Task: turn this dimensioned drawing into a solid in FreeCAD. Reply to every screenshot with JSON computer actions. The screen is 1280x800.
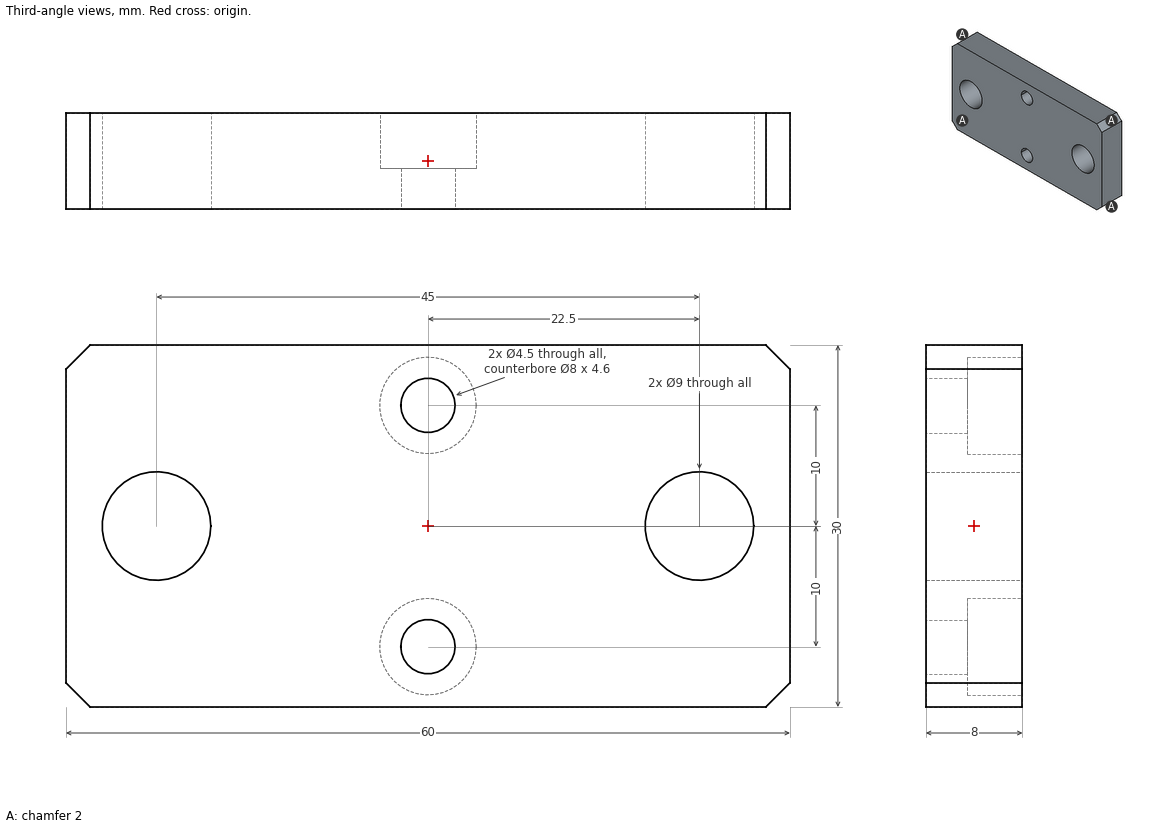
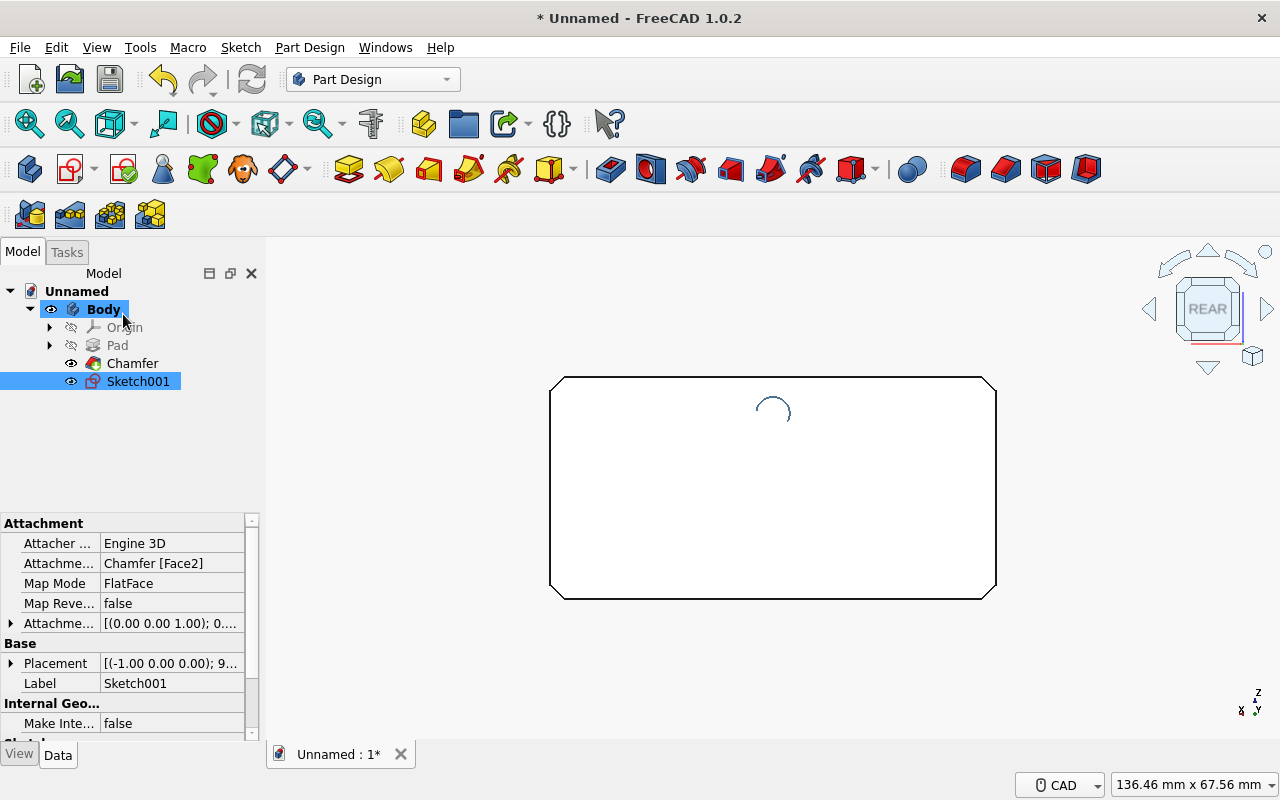
{"action": "left_click", "coordinate": [652, 170]}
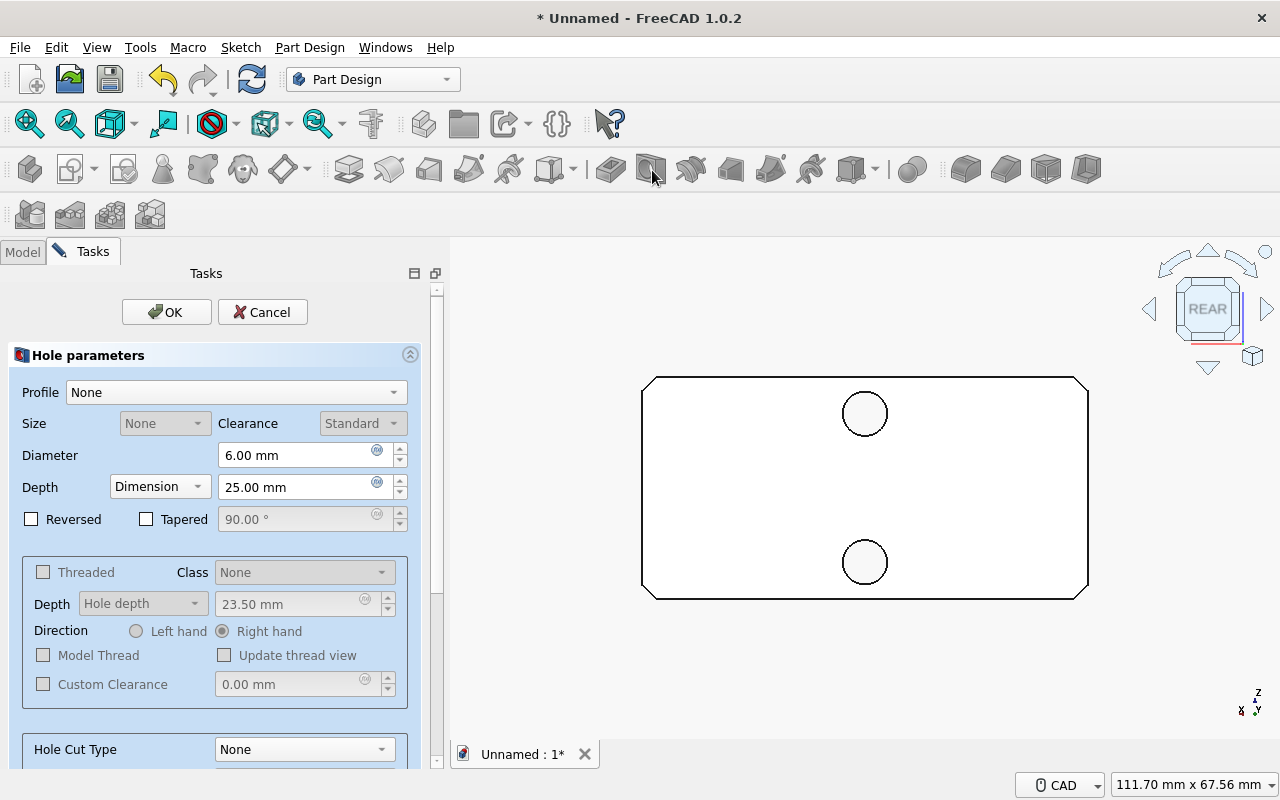
{"action": "triple_click", "coordinate": [305, 455]}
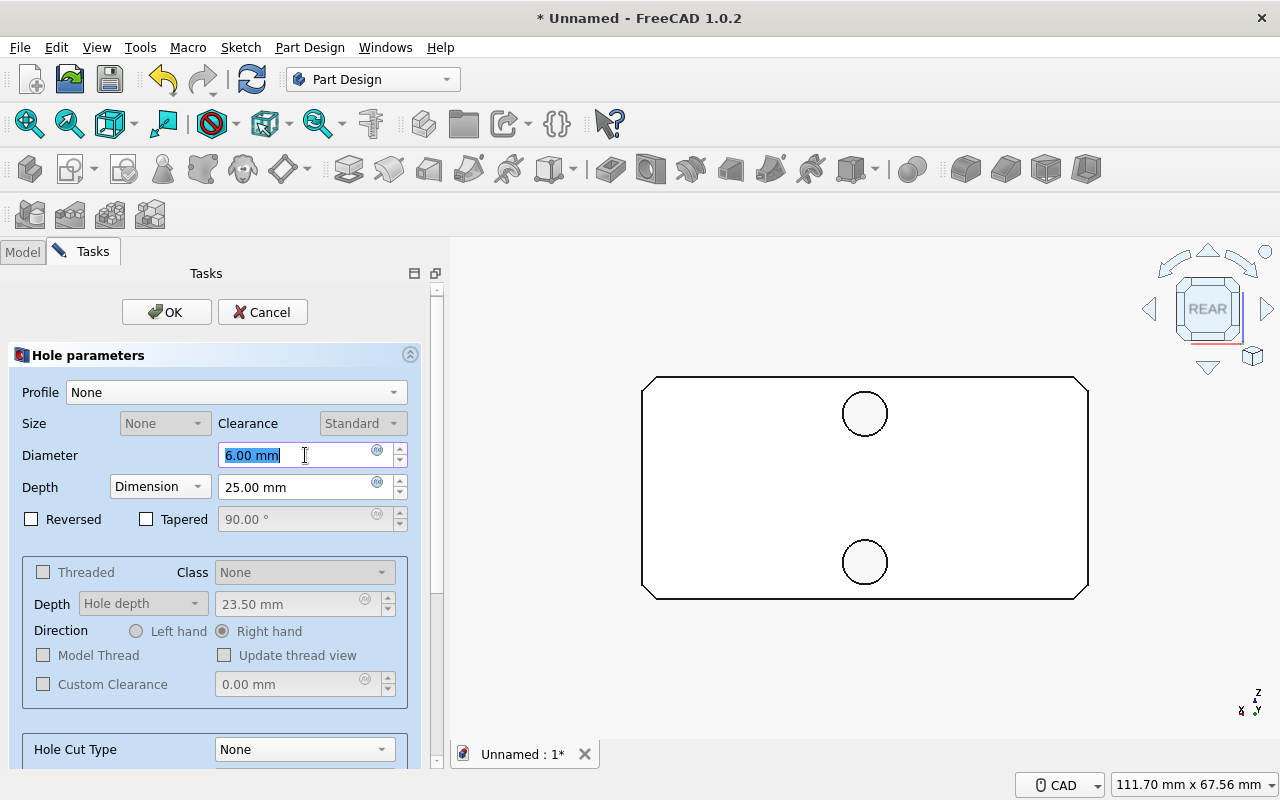
{"action": "type", "text": "4.5"}
{"action": "key", "text": "Tab"}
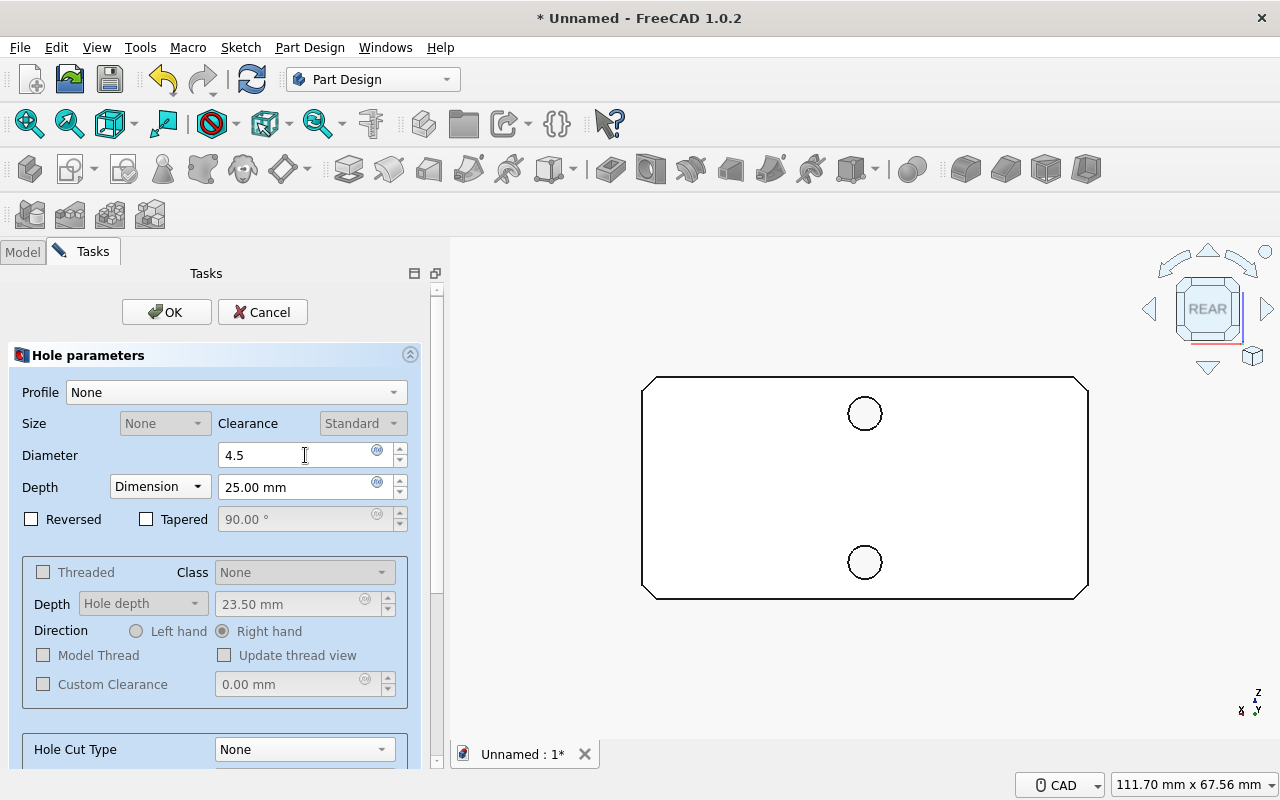
{"action": "left_click", "coordinate": [161, 486]}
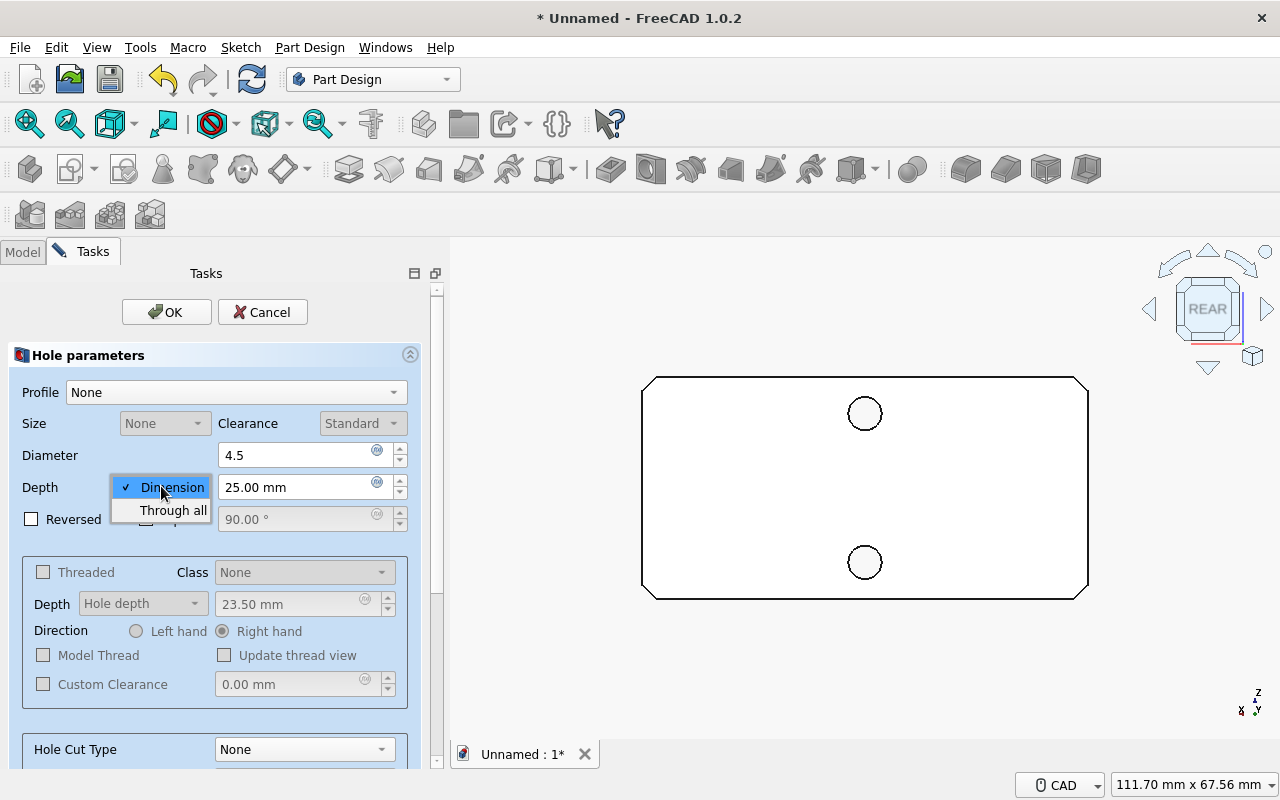
{"action": "left_click", "coordinate": [160, 510]}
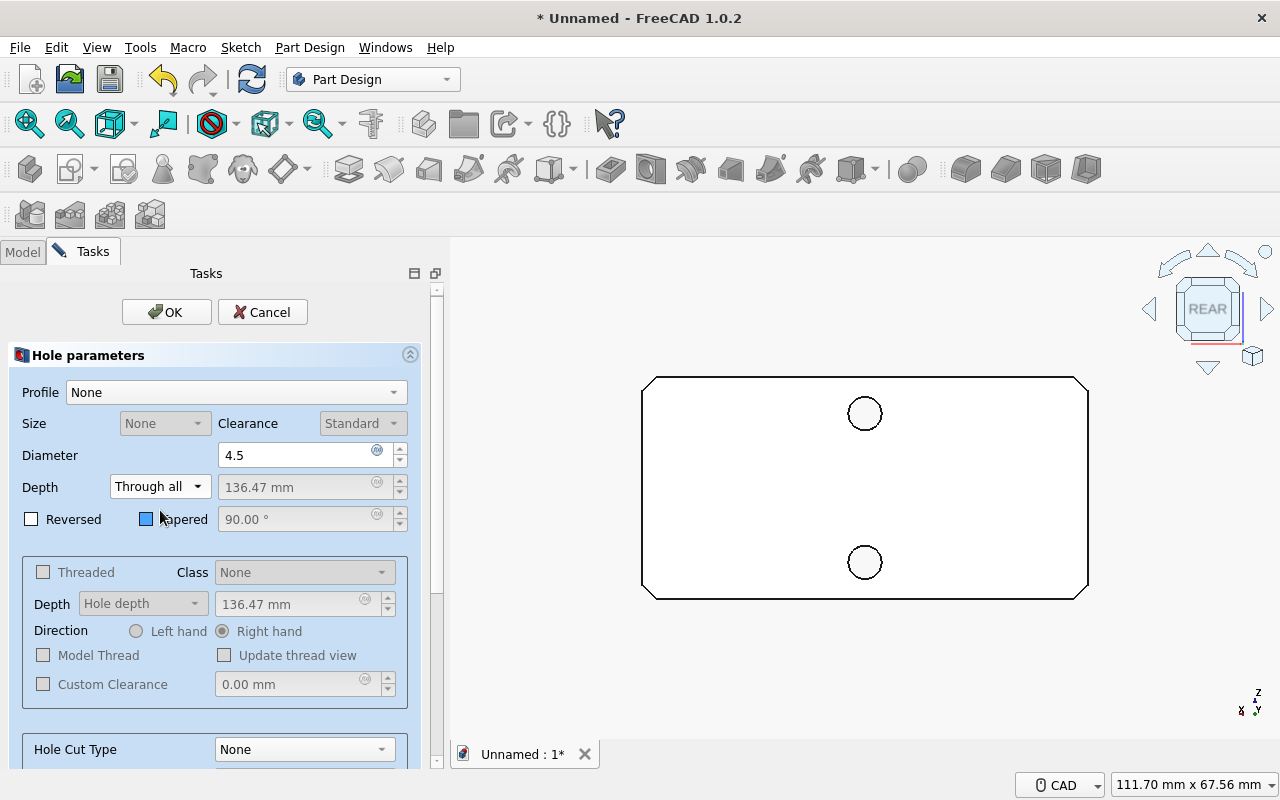
{"action": "left_click", "coordinate": [306, 750]}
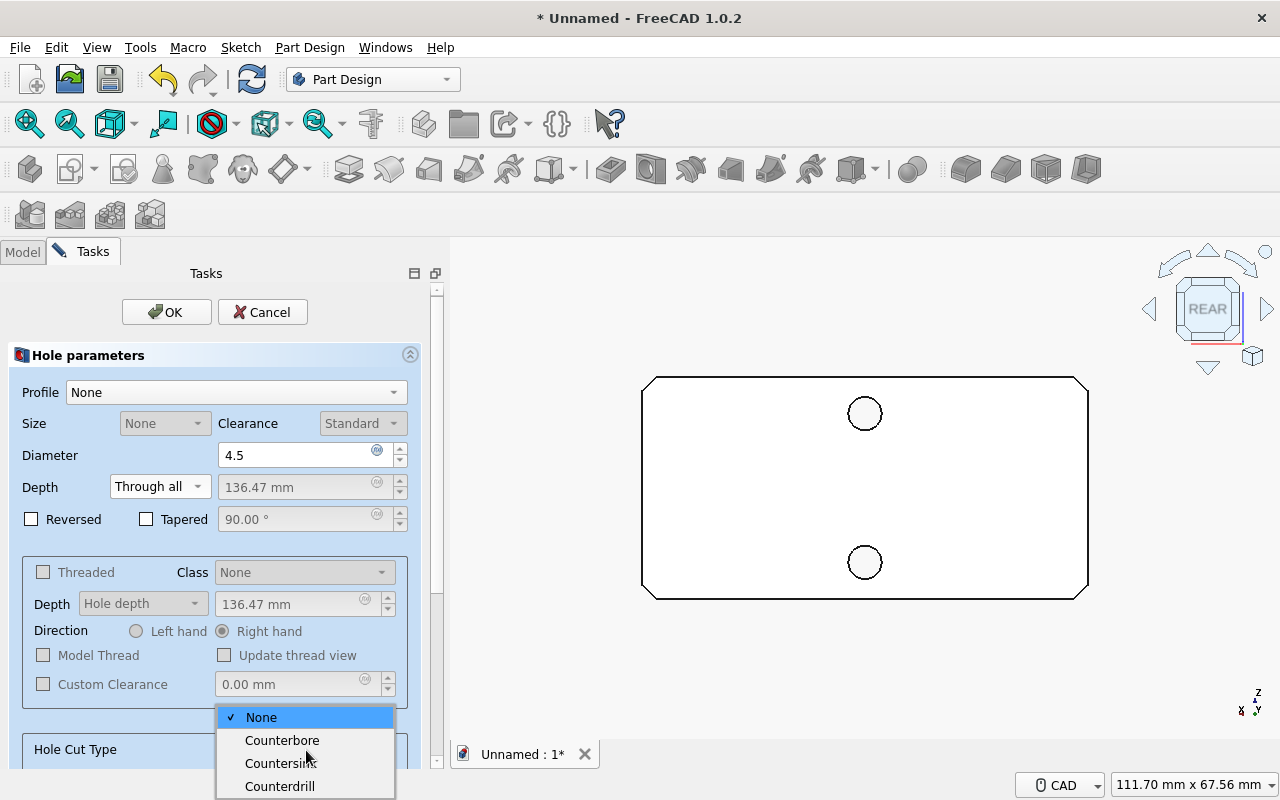
{"action": "left_click", "coordinate": [304, 740]}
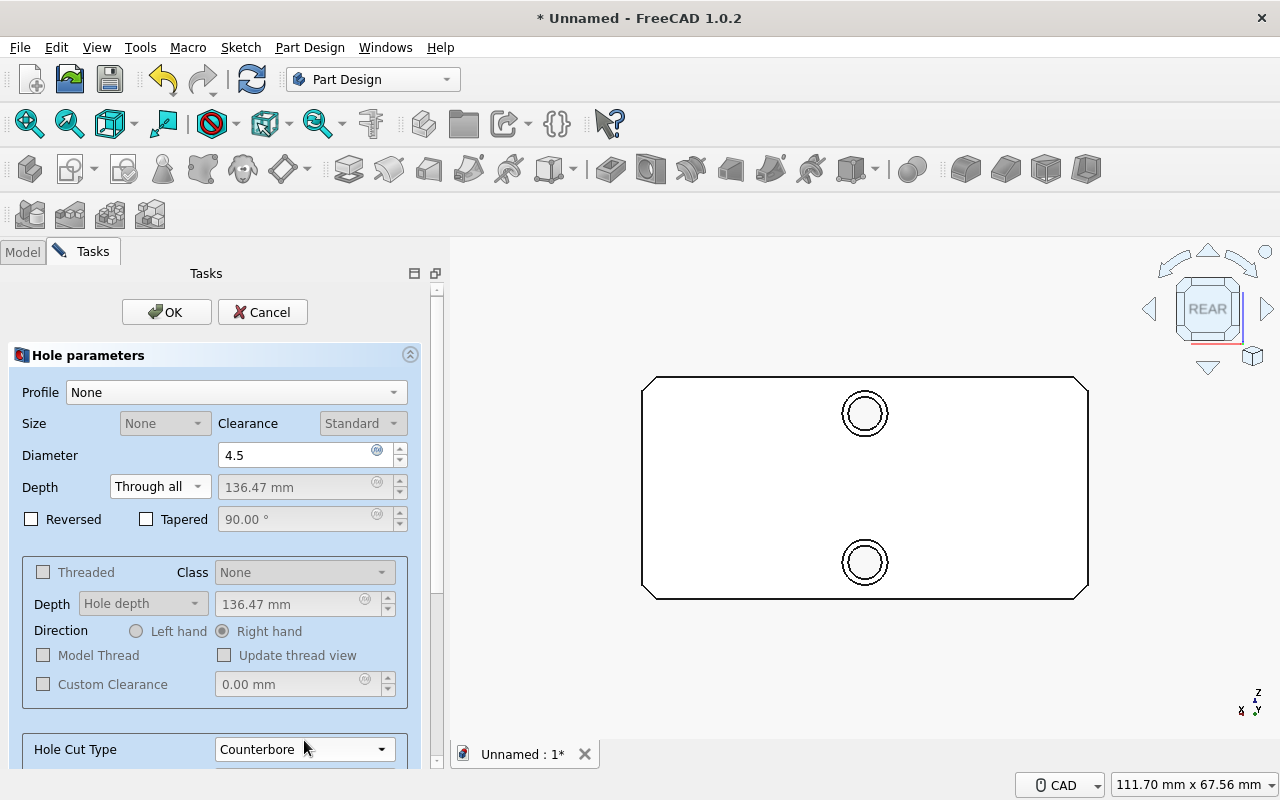
{"action": "scroll", "coordinate": [437, 526], "scroll_direction": "down", "scroll_amount": 2}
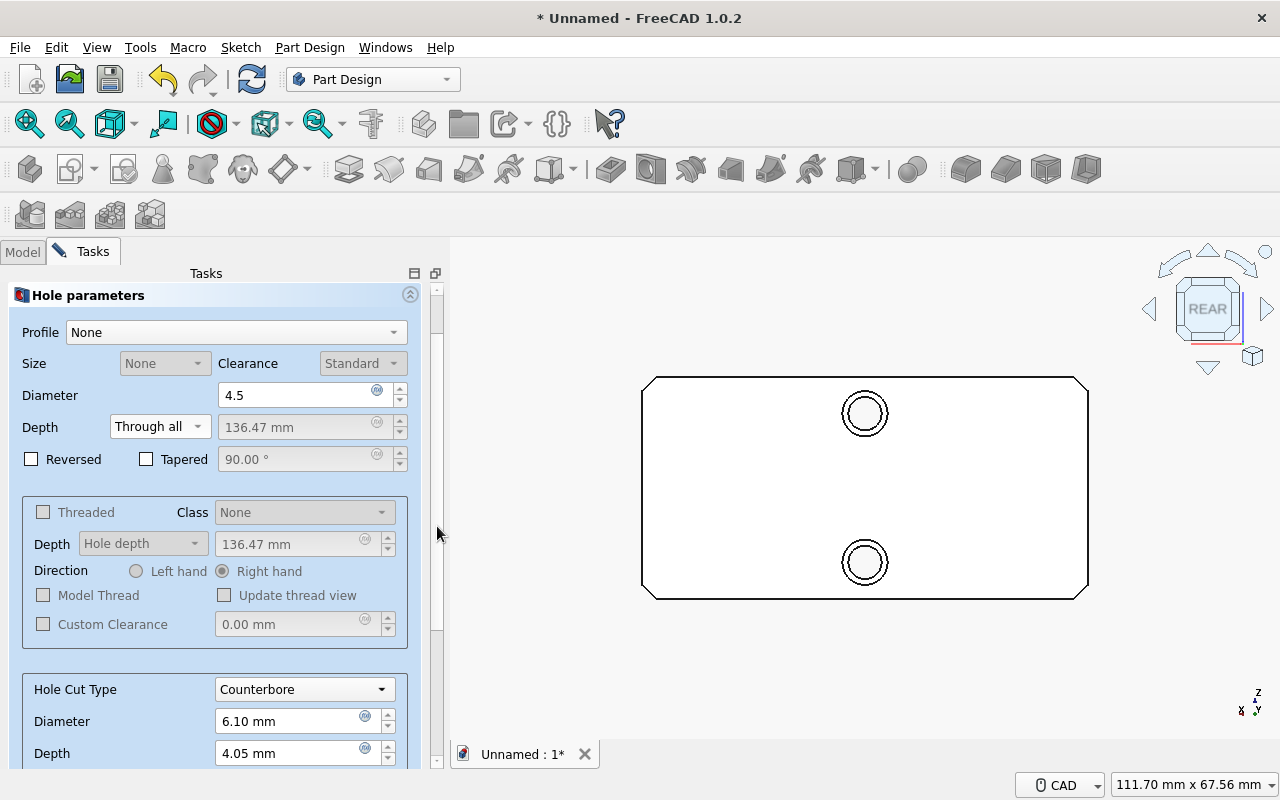
{"action": "triple_click", "coordinate": [298, 661]}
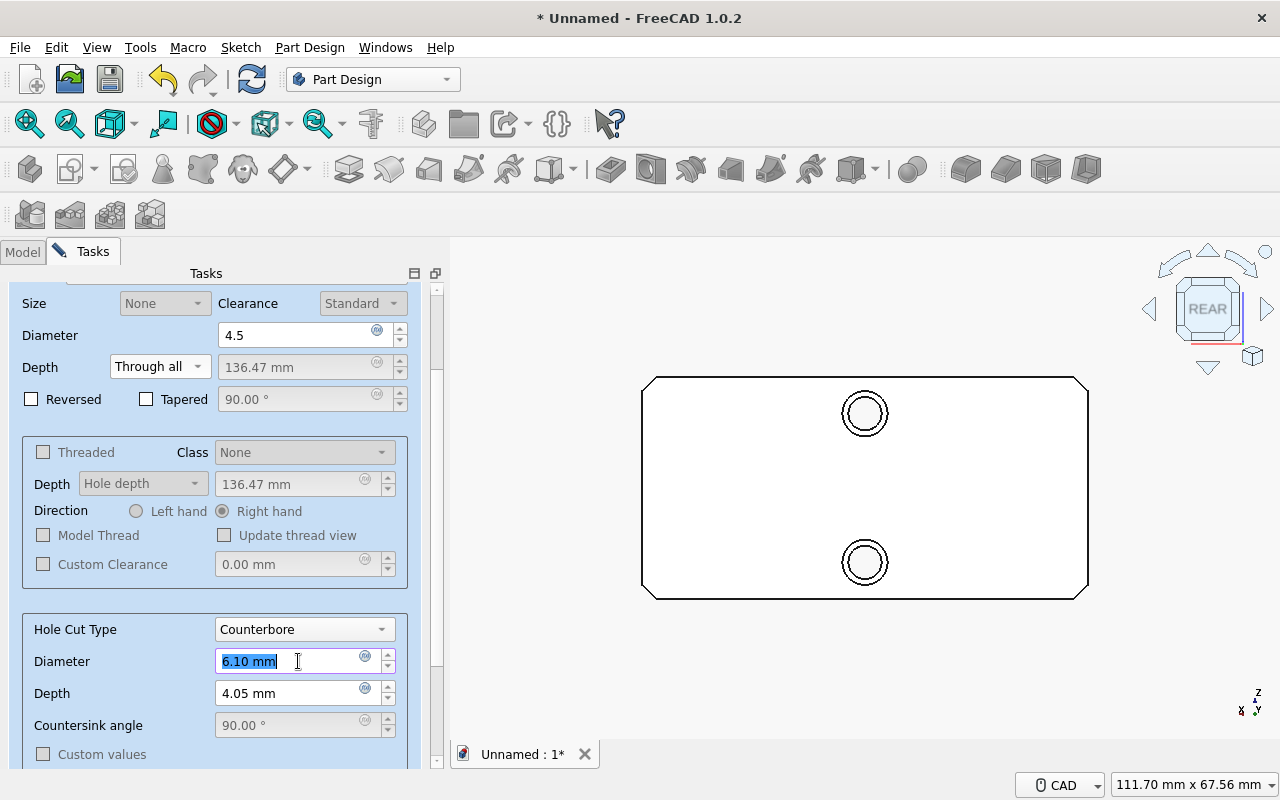
{"action": "type", "text": "8"}
{"action": "key", "text": "Tab"}